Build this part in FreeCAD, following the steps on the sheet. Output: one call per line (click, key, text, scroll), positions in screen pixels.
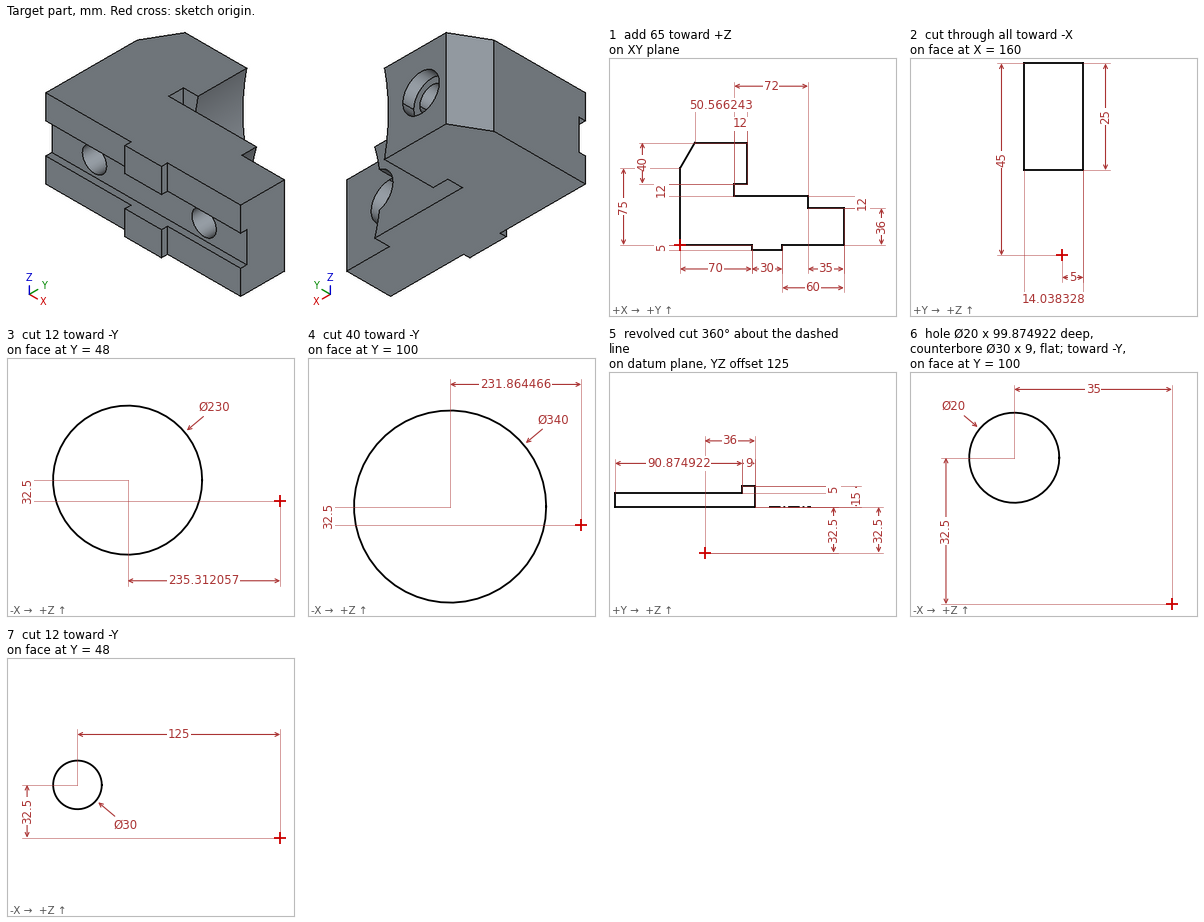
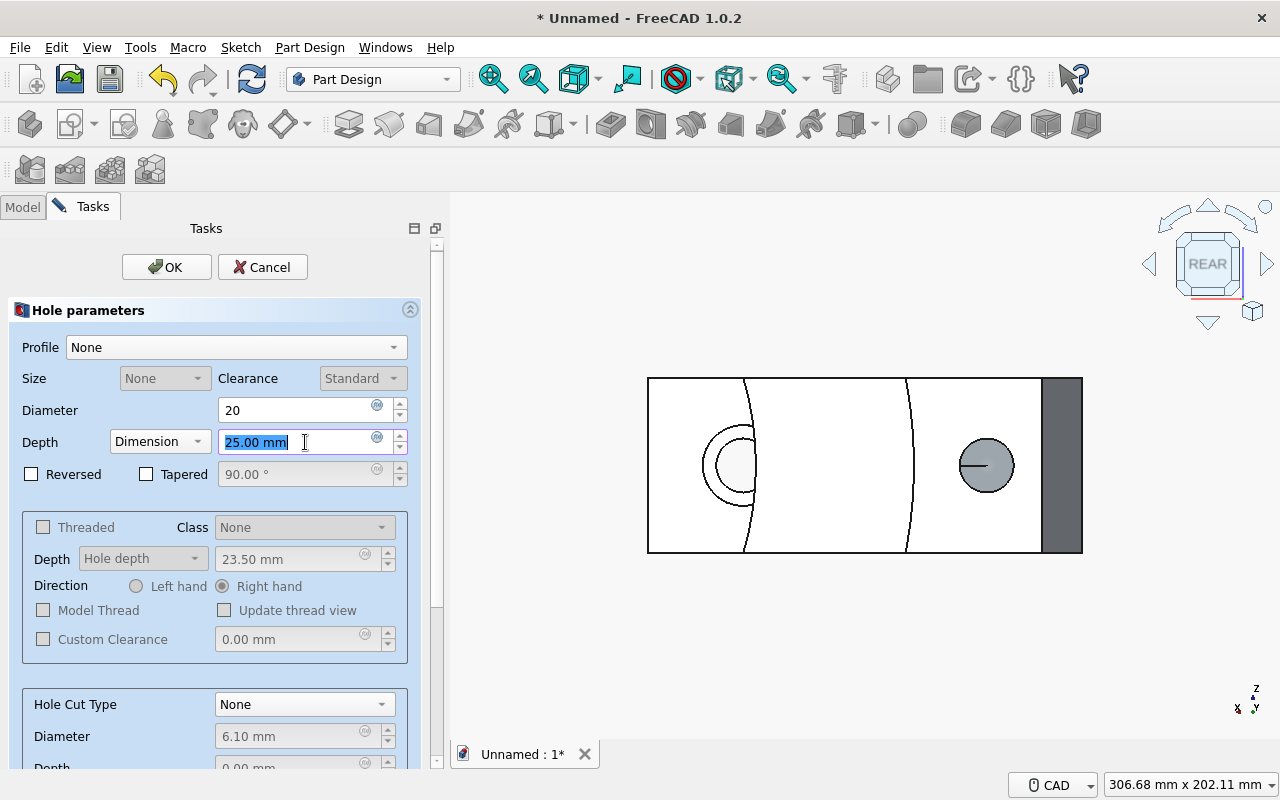
text(99.874922)
key(Tab)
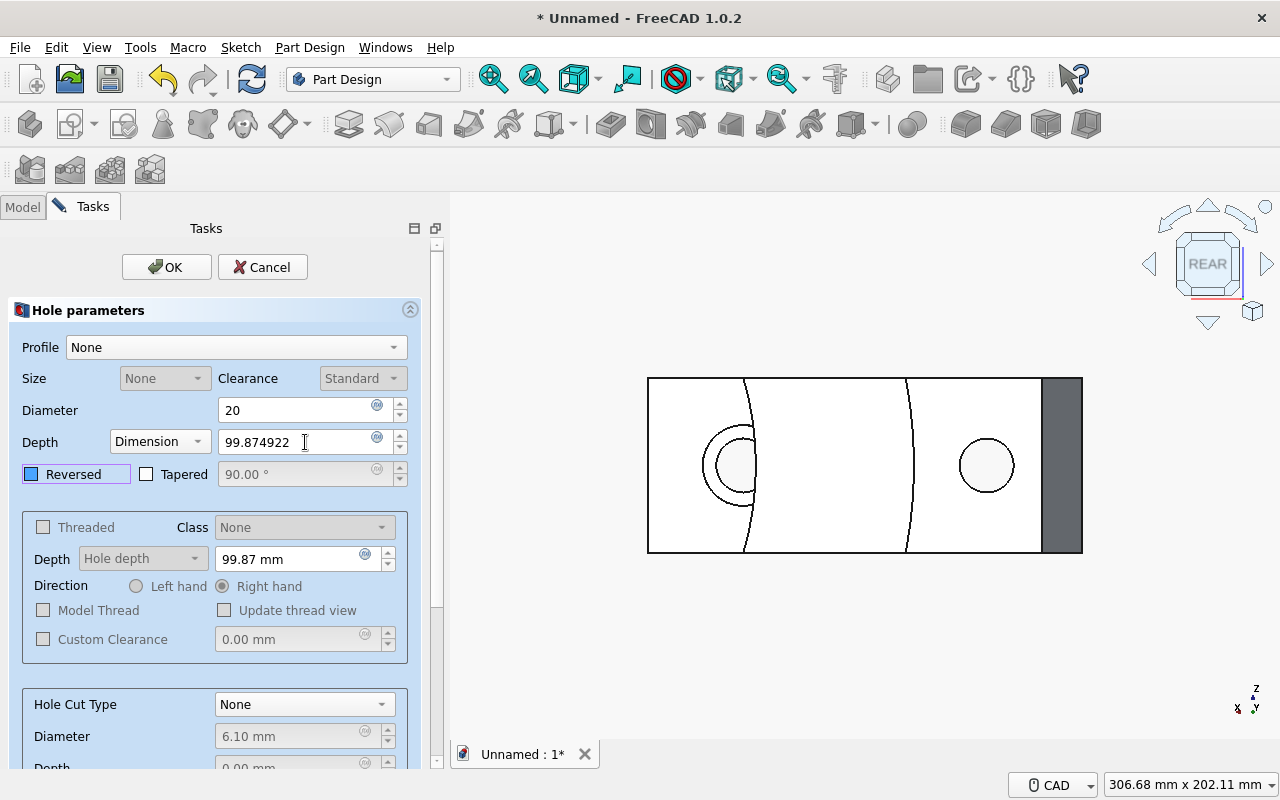
click(306, 704)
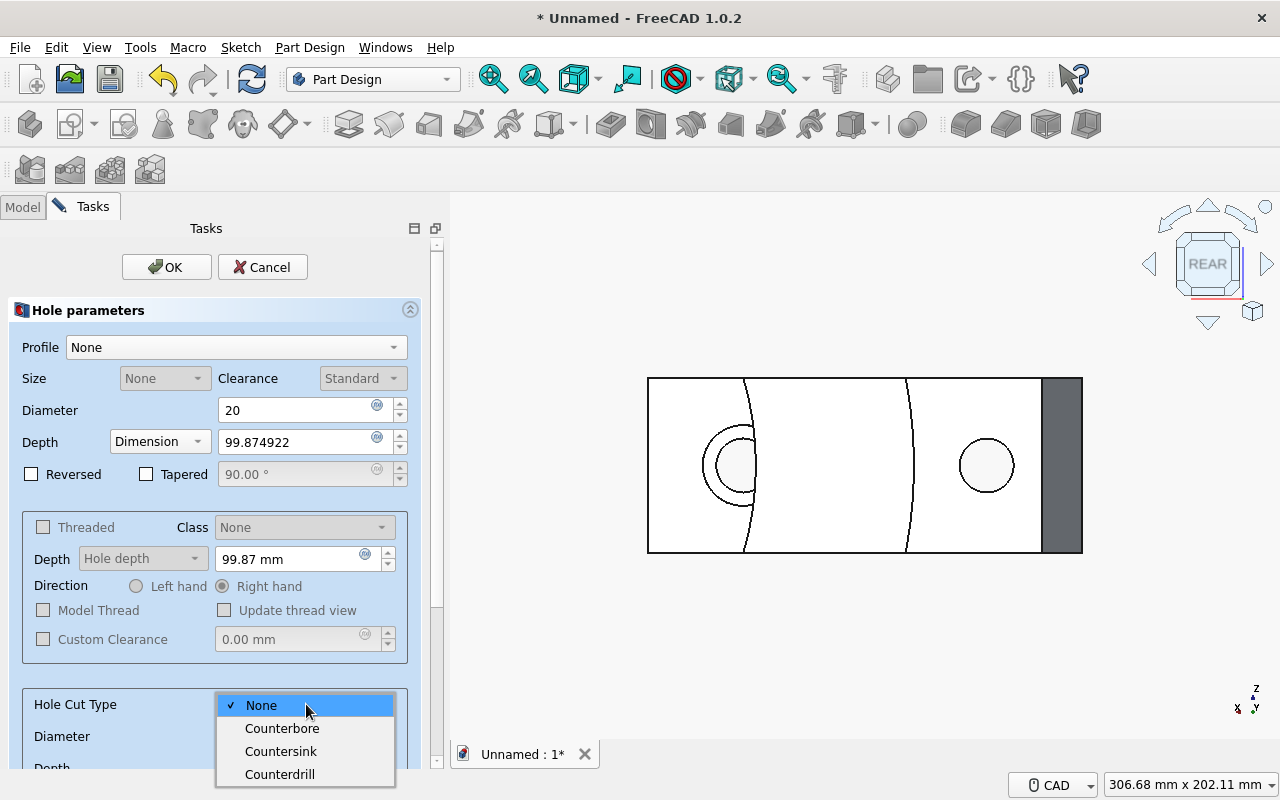
click(304, 728)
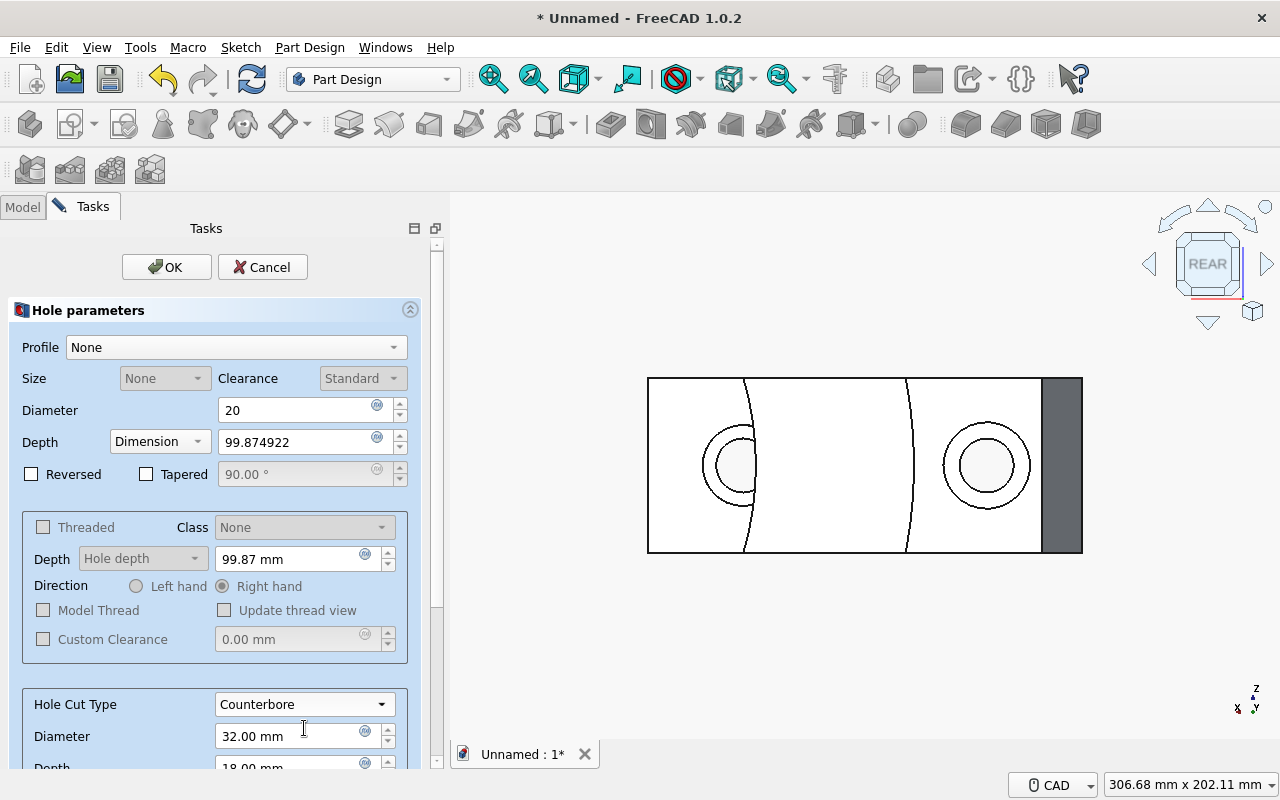
triple_click(298, 736)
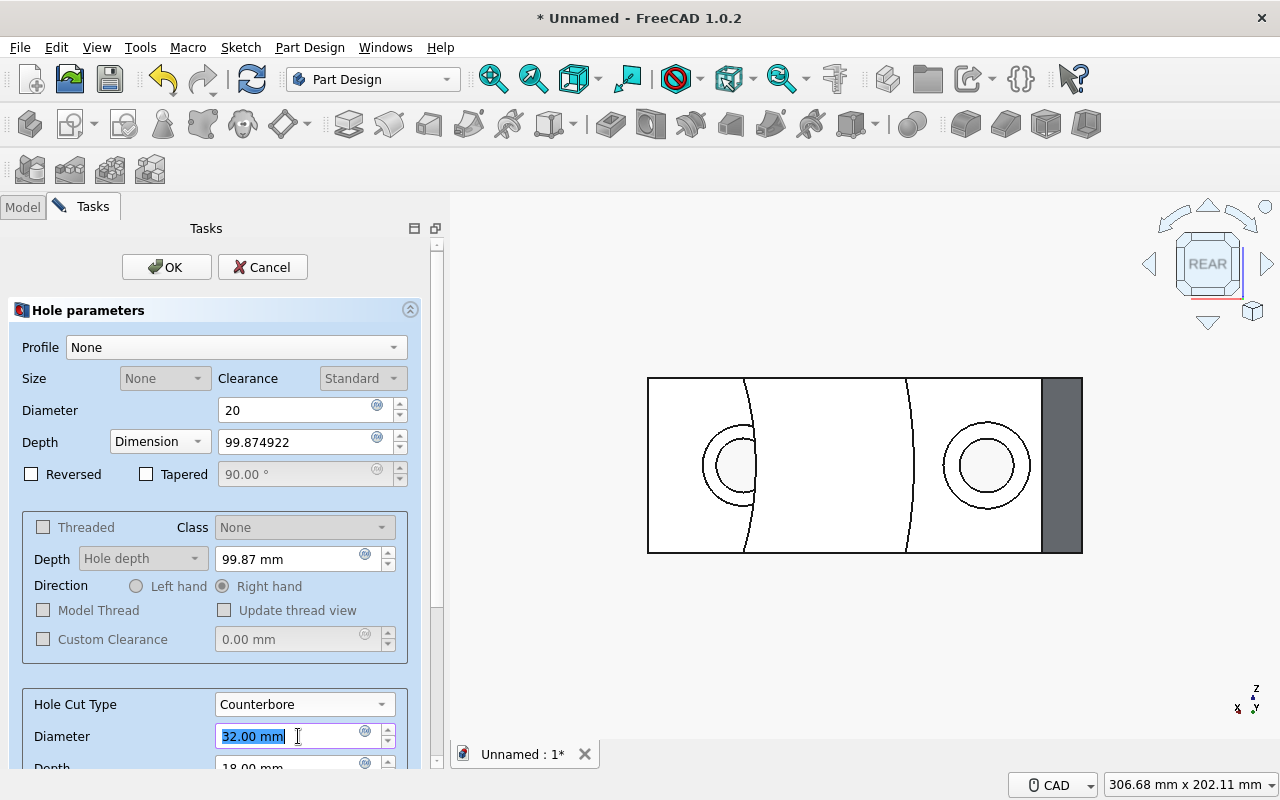
text(30)
key(Tab)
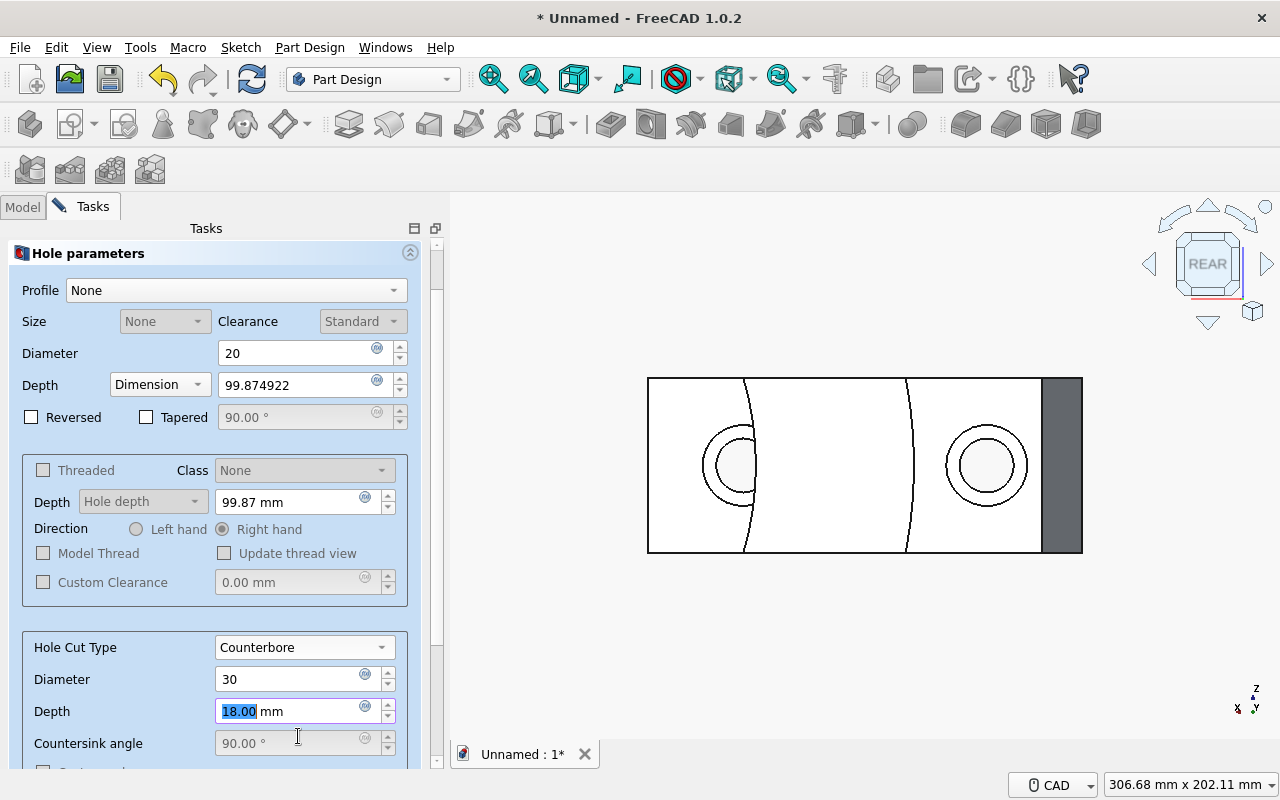
text(9)
key(Tab)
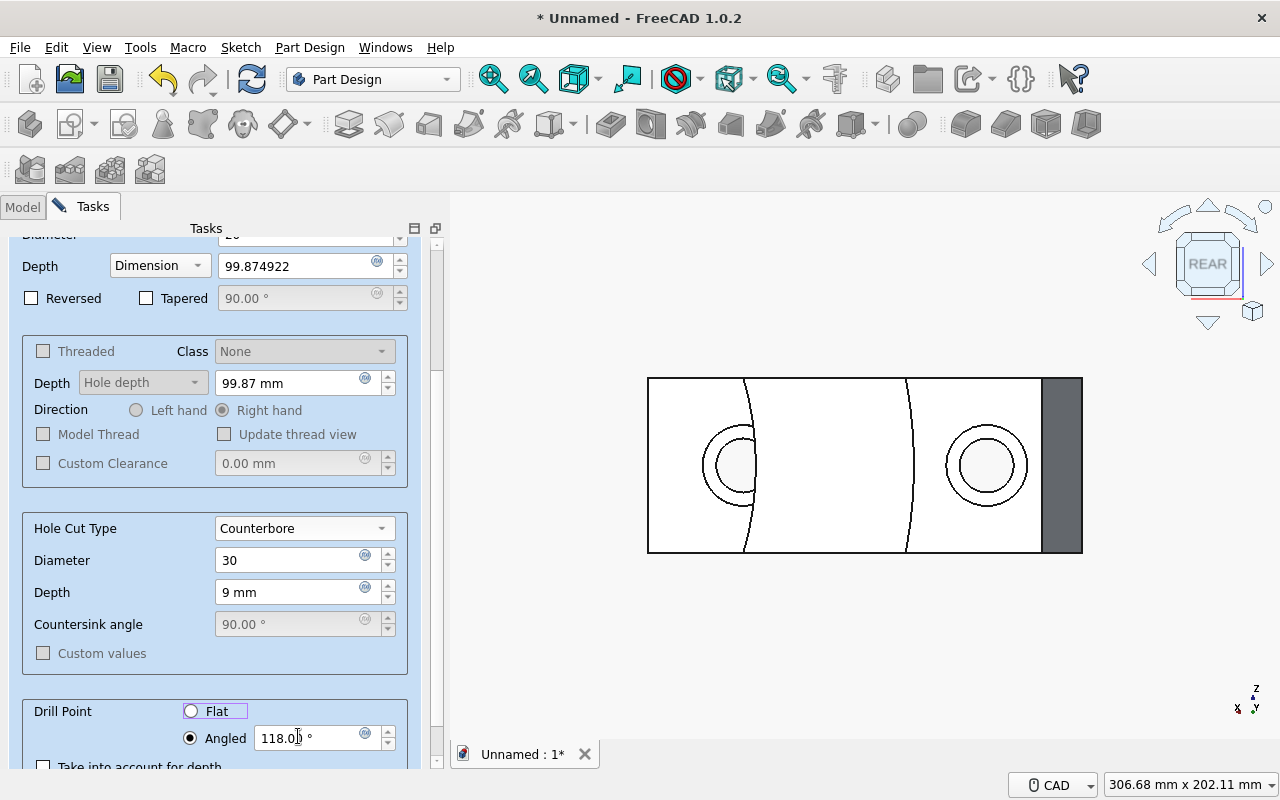
click(191, 711)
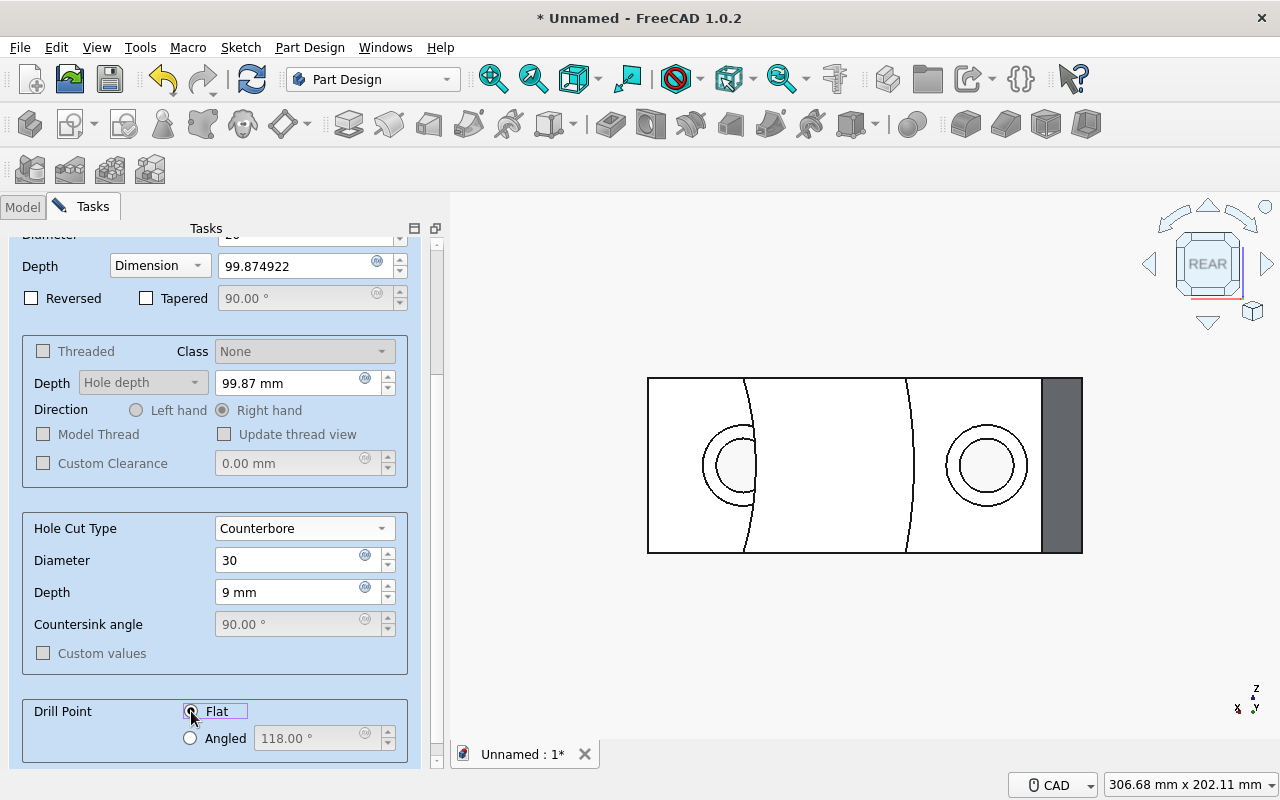
scroll(437, 503, up, 4)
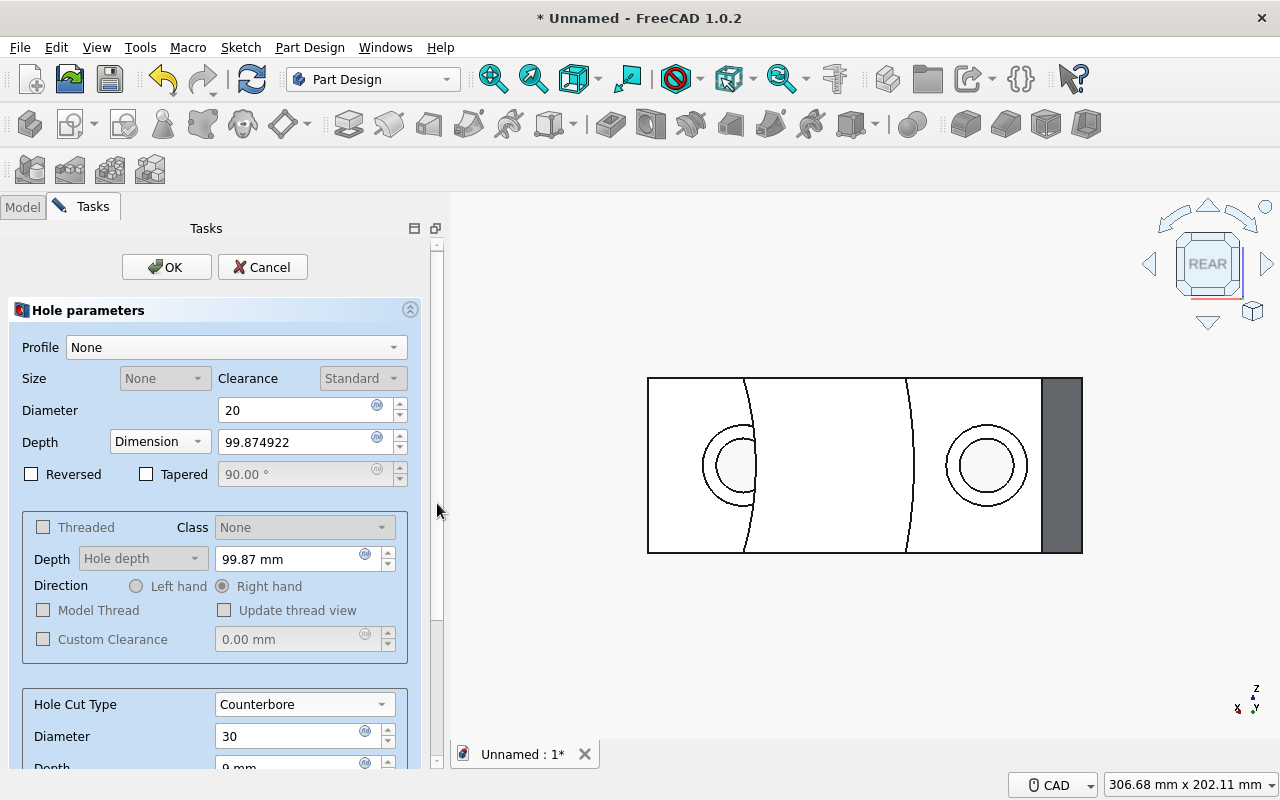
click(167, 267)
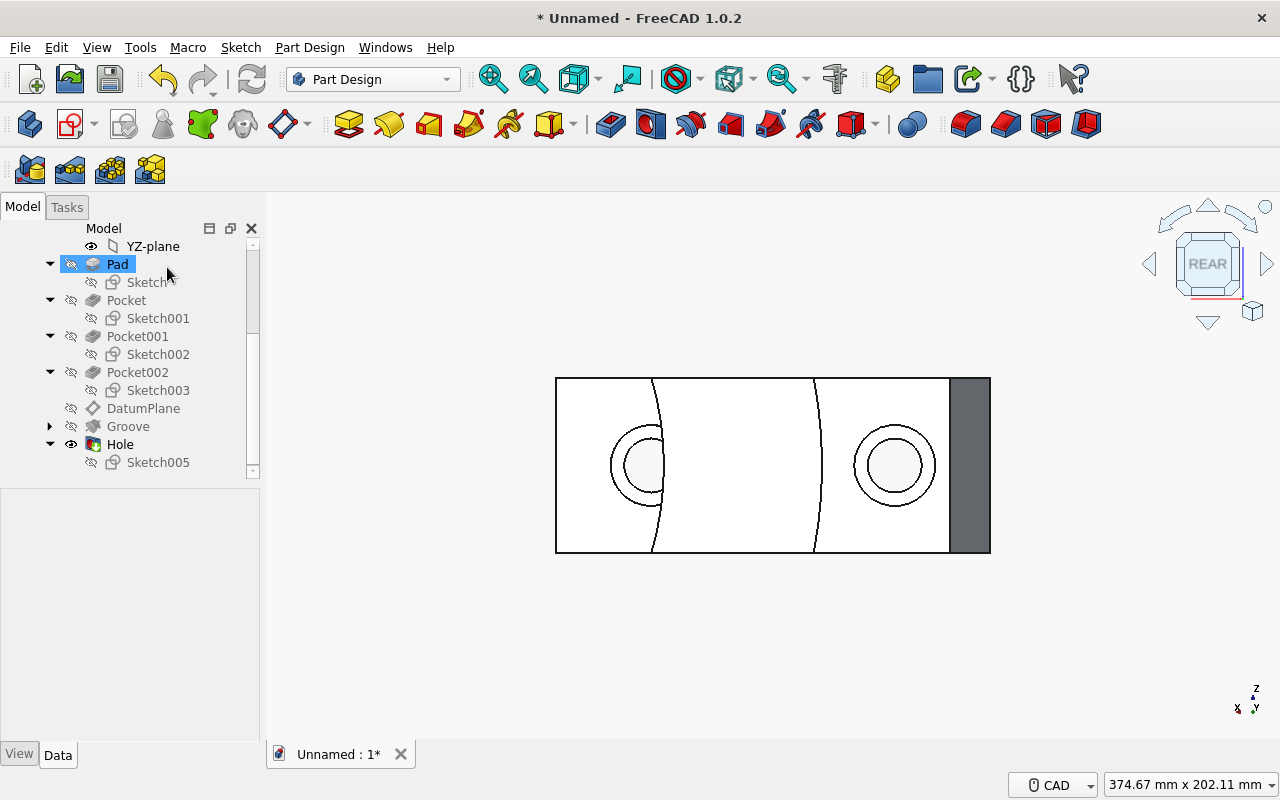
click(494, 80)